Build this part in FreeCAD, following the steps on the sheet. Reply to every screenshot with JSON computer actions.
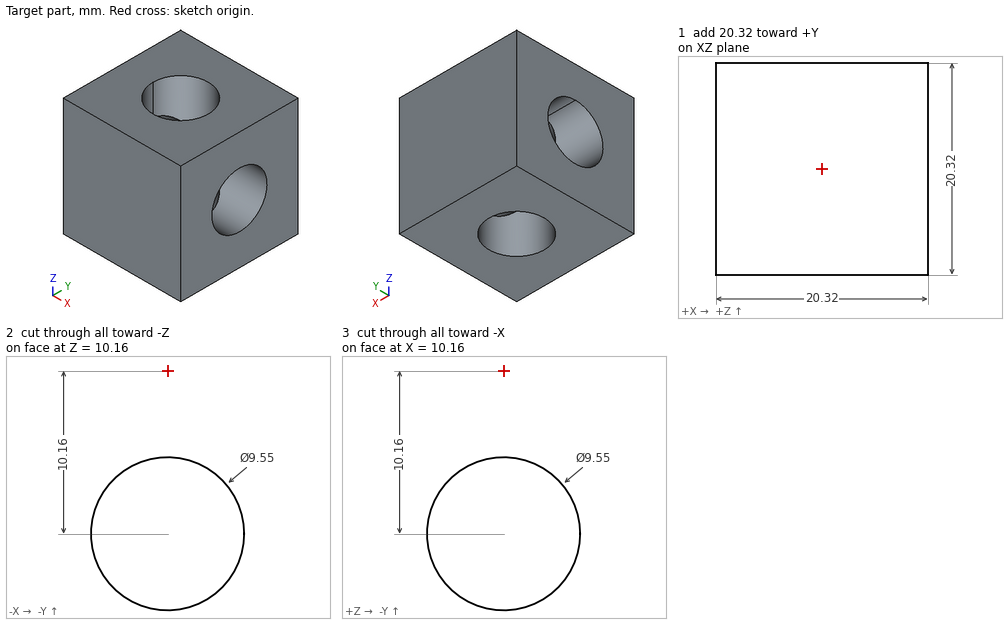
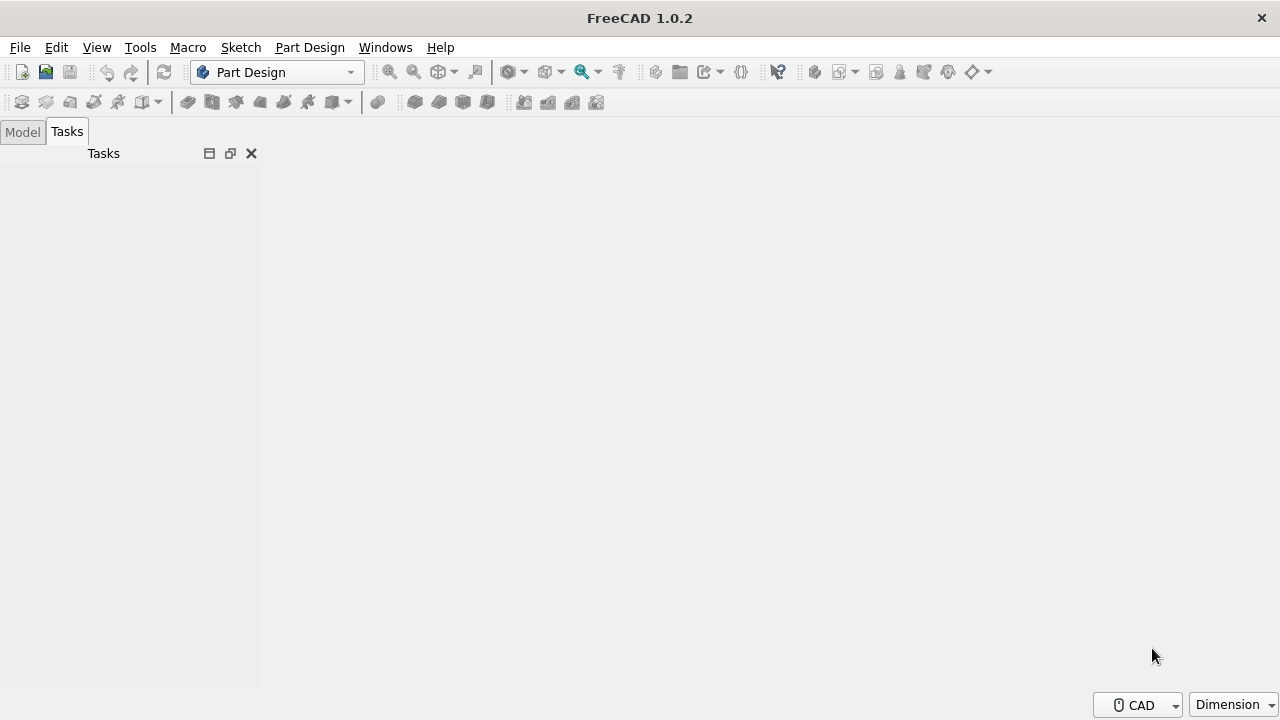
{"action": "left_click", "coordinate": [22, 72]}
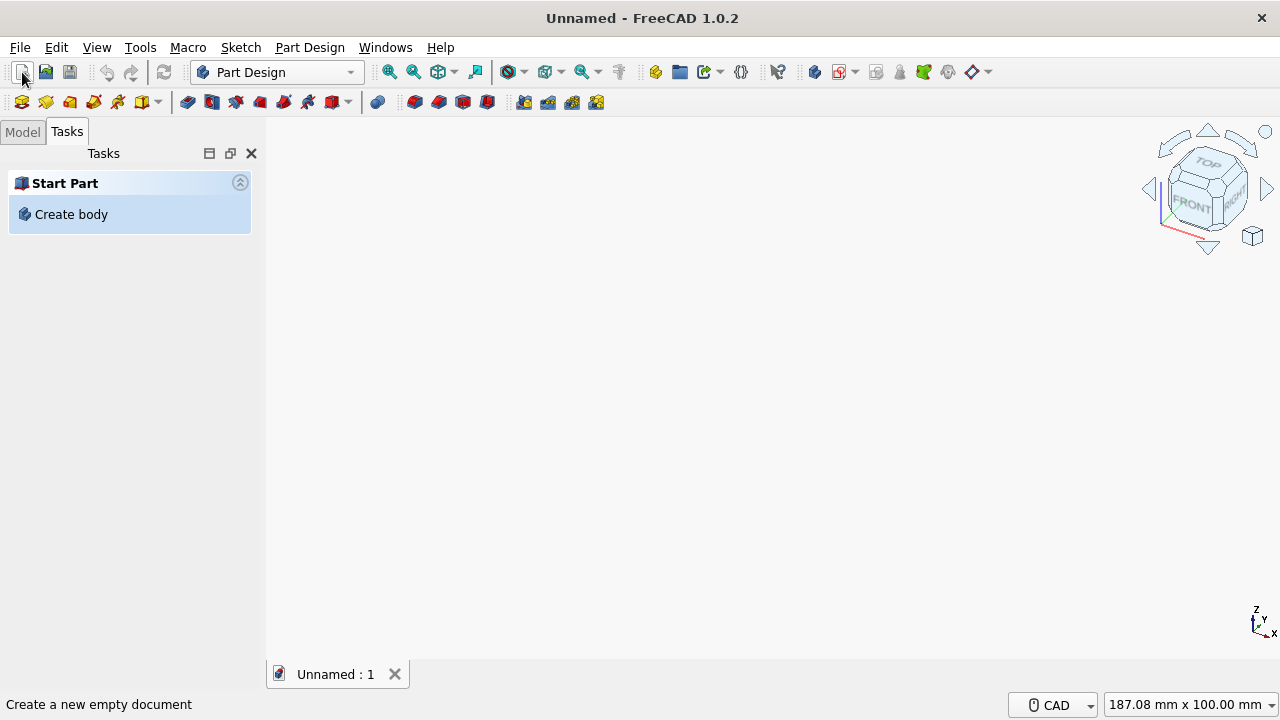
{"action": "left_click", "coordinate": [840, 72]}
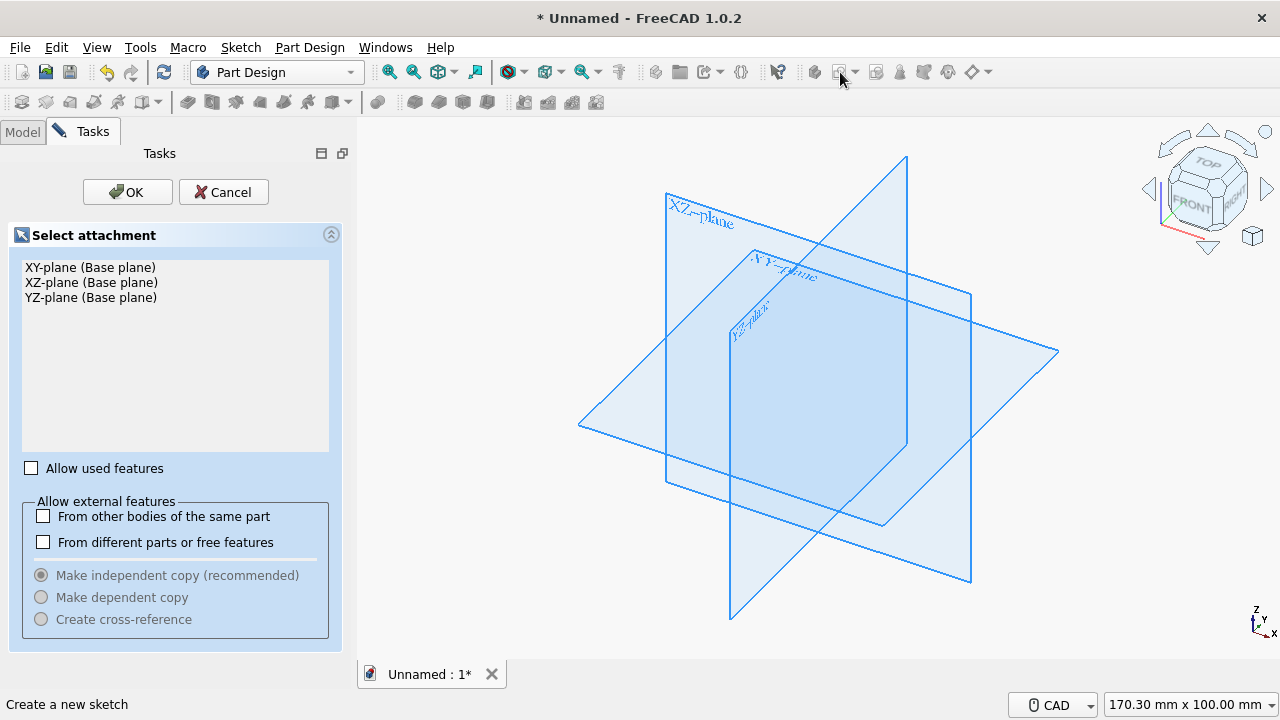
{"action": "left_click", "coordinate": [82, 282]}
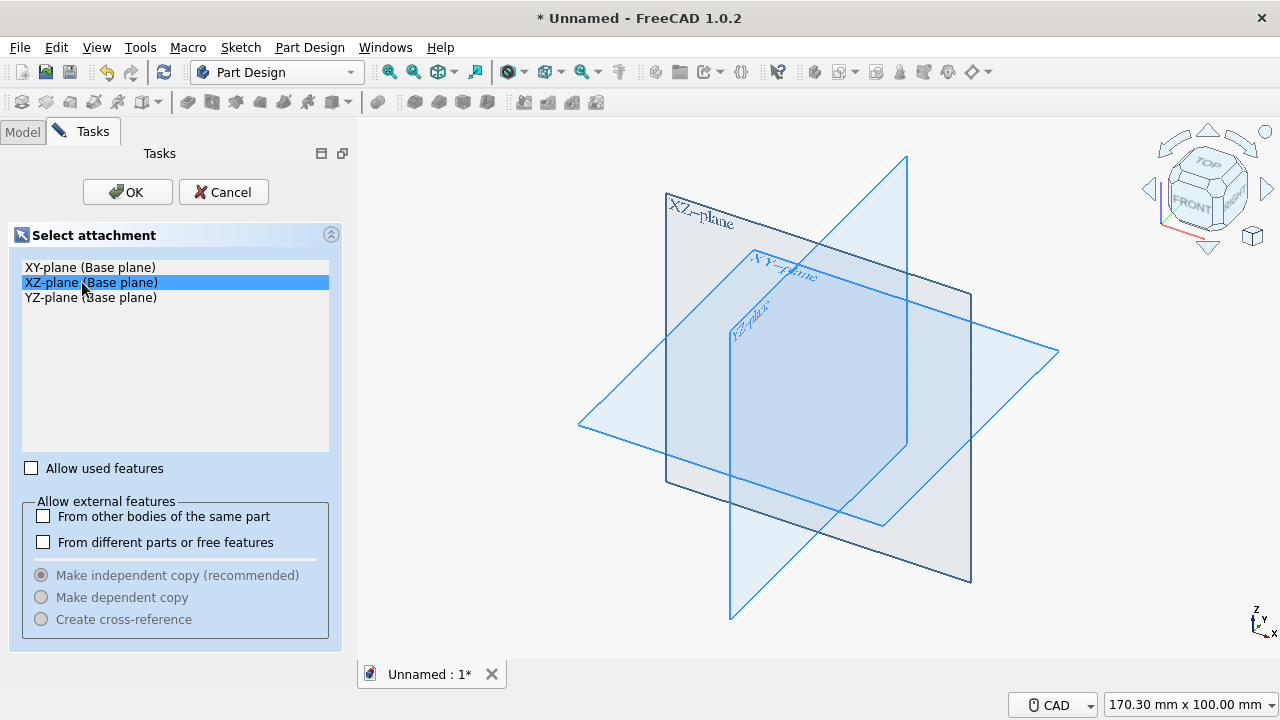
{"action": "left_click", "coordinate": [128, 192]}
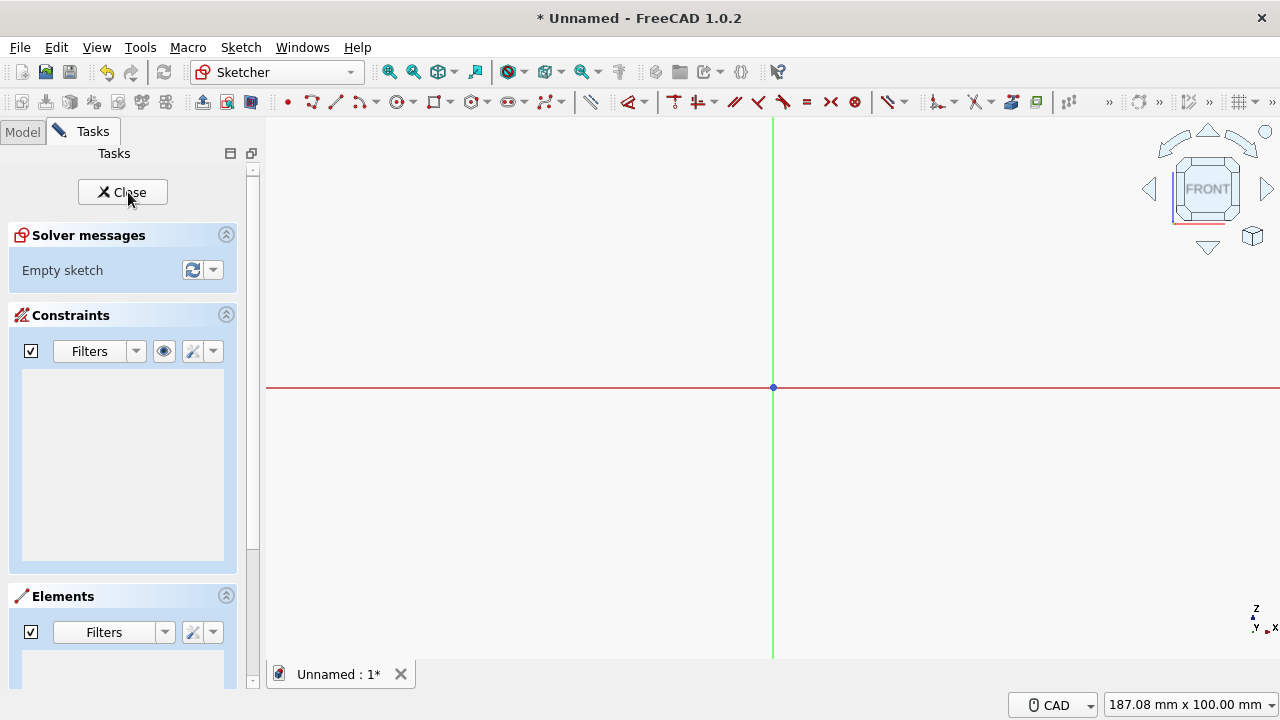
{"action": "scroll", "coordinate": [803, 388], "scroll_direction": "up", "scroll_amount": 6}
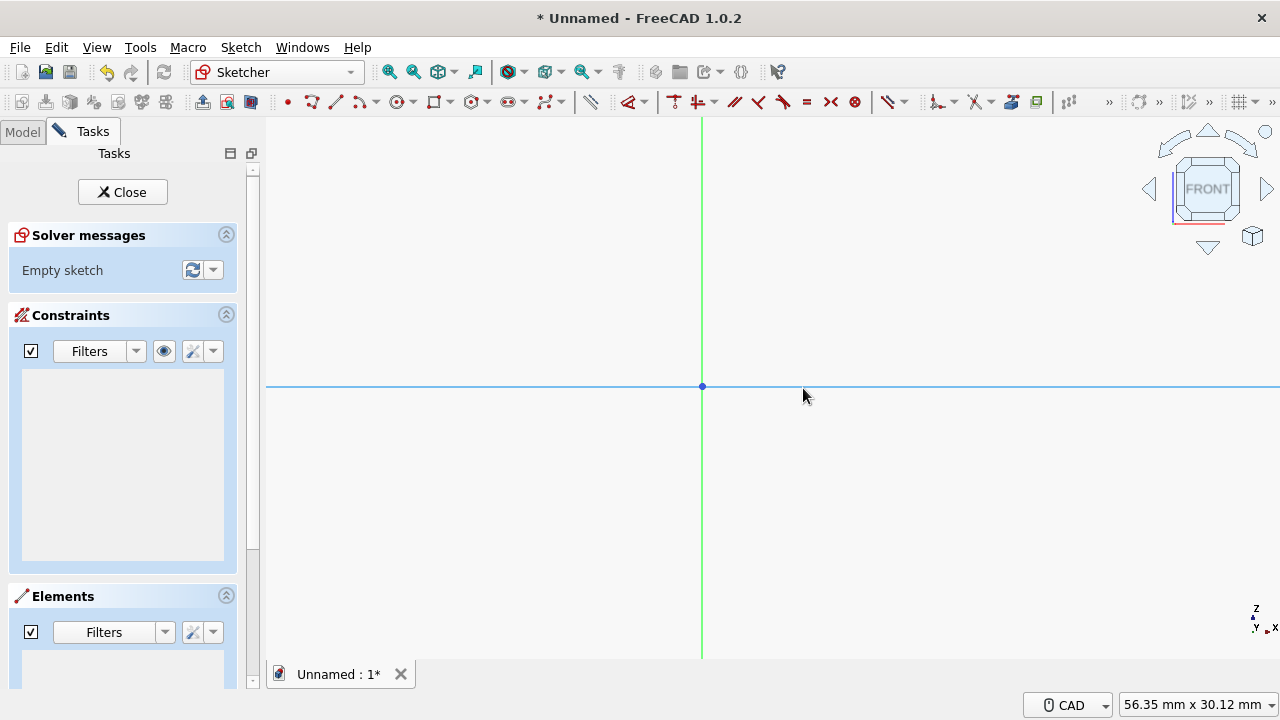
{"action": "key", "text": "g v"}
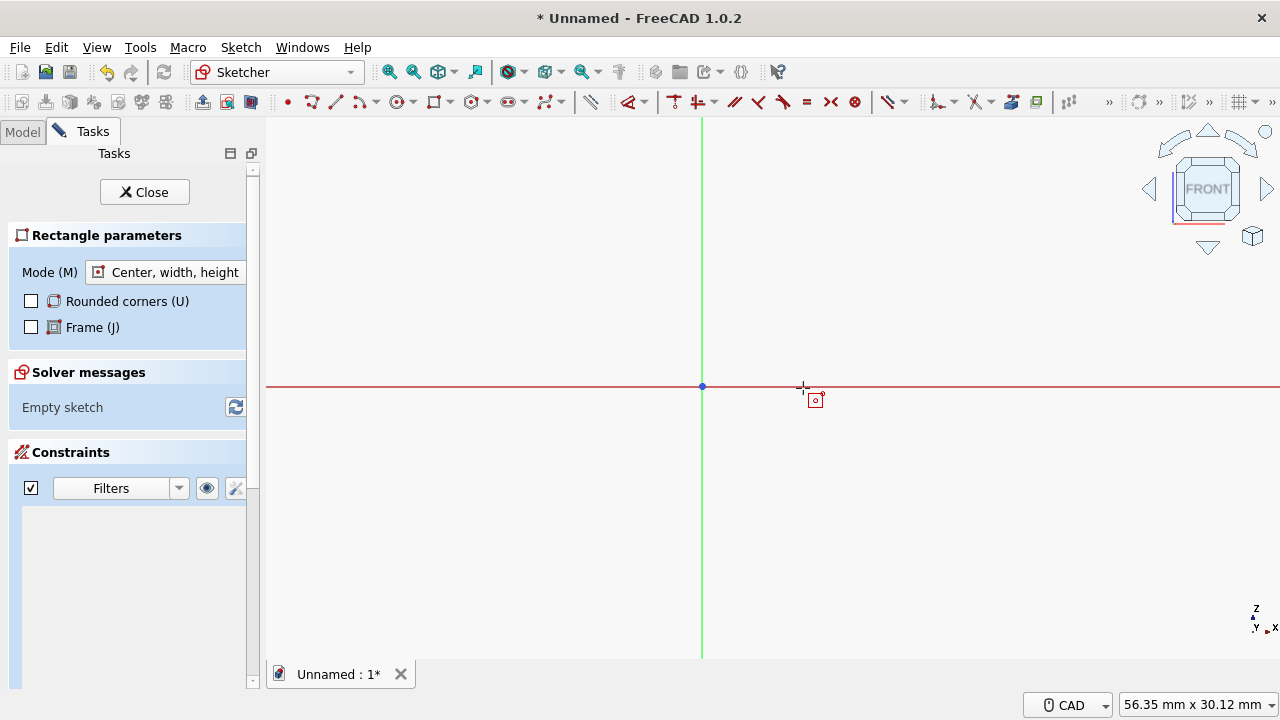
{"action": "left_click", "coordinate": [702, 387]}
{"action": "mouse_move", "coordinate": [885, 204]}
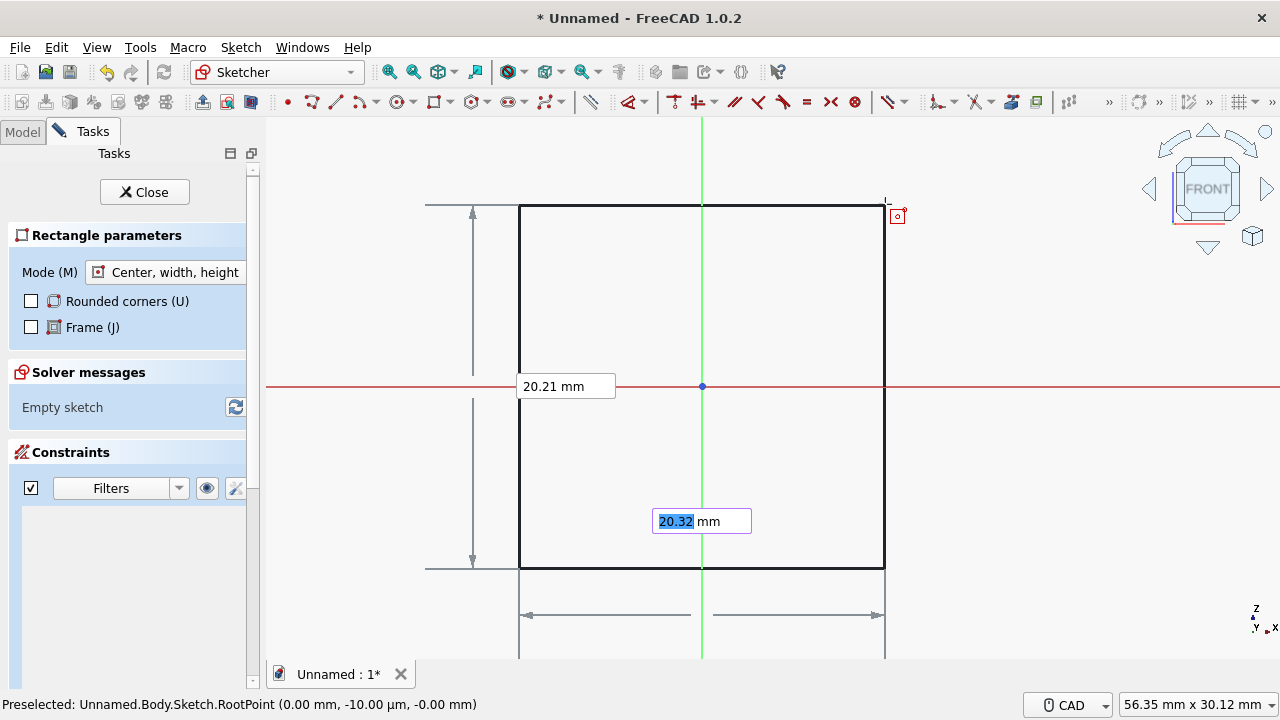
{"action": "type", "text": "20.32"}
{"action": "key", "text": "Tab"}
{"action": "type", "text": "20.32"}
{"action": "key", "text": "Return"}
{"action": "key", "text": "Escape"}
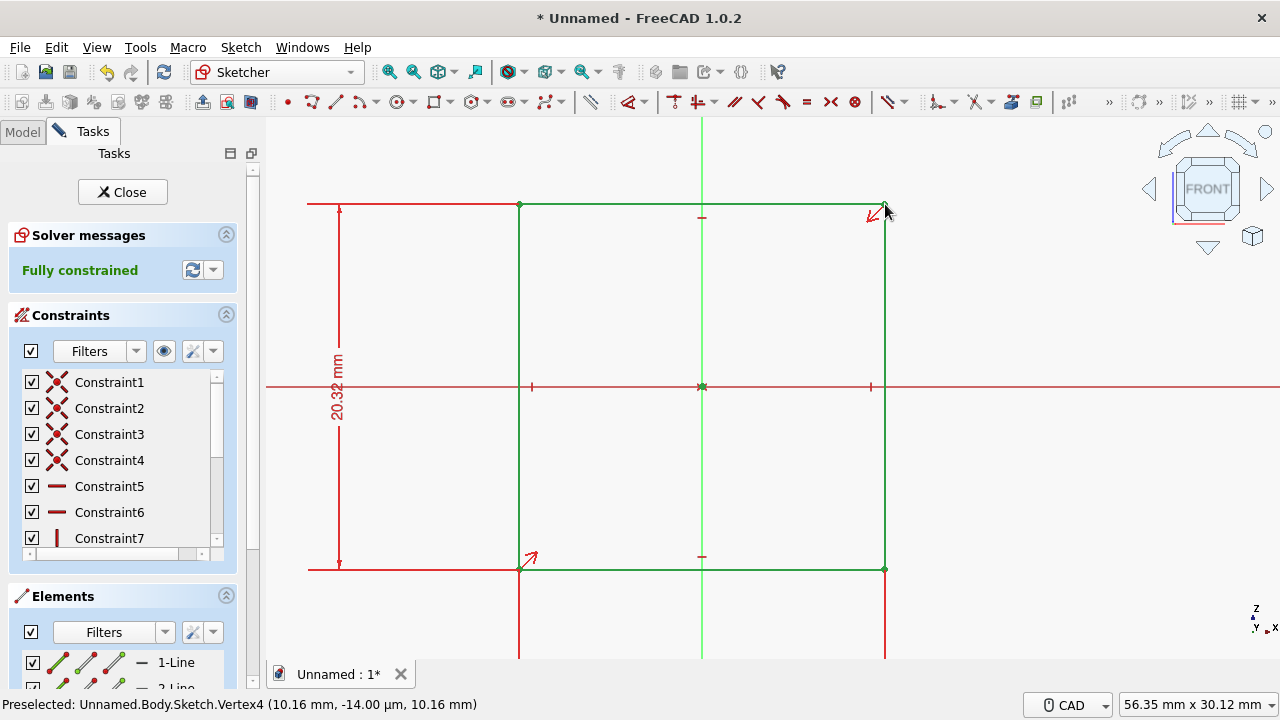
{"action": "left_click", "coordinate": [123, 192]}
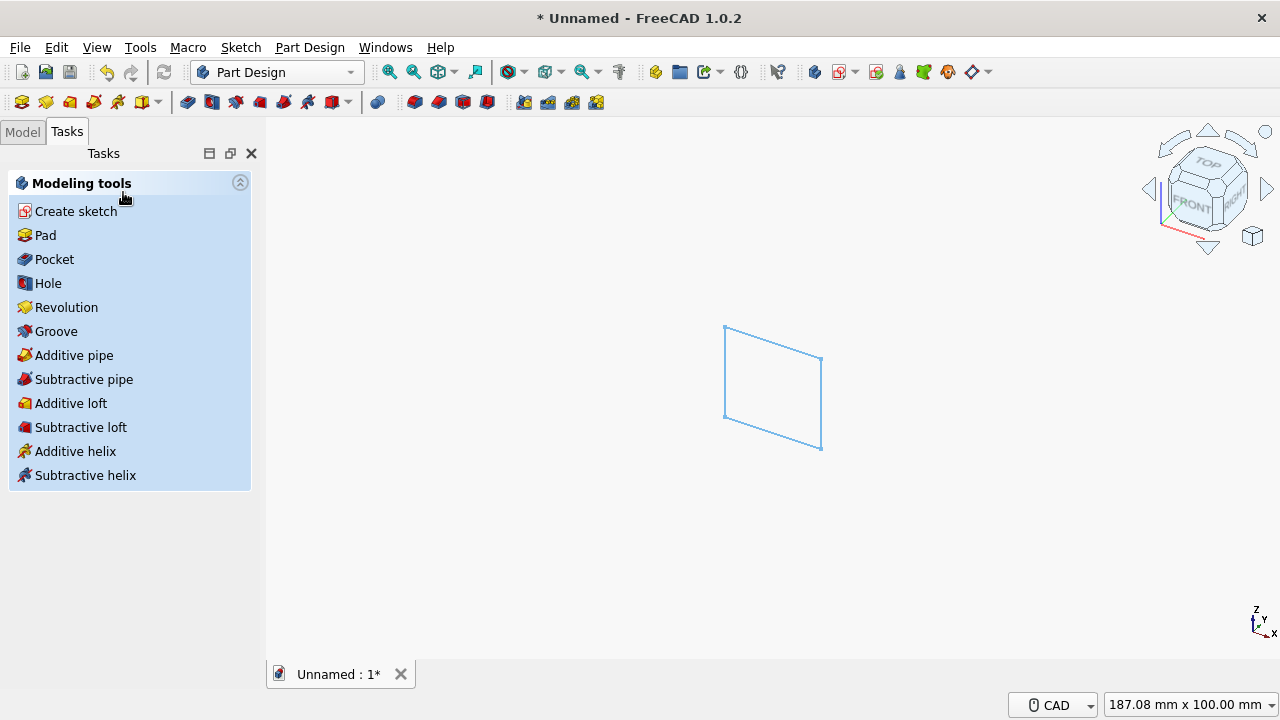
{"action": "left_click", "coordinate": [22, 102]}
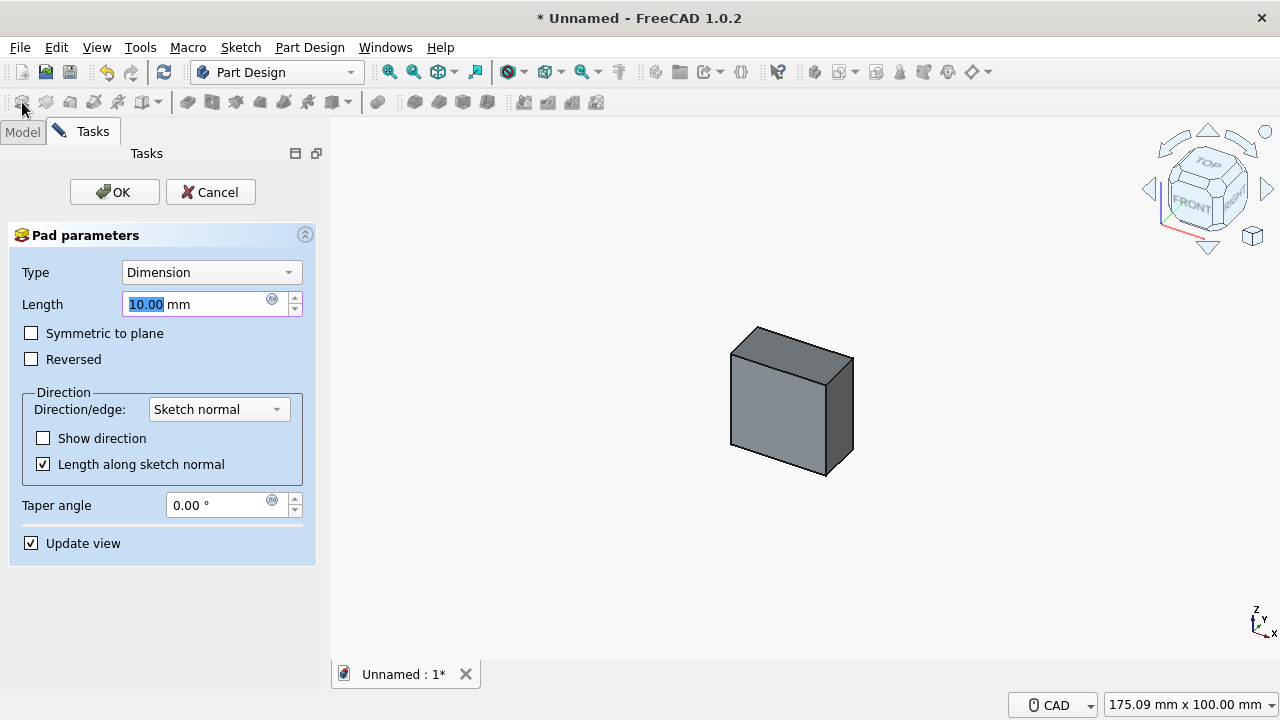
{"action": "type", "text": "20.32"}
{"action": "key", "text": "Tab"}